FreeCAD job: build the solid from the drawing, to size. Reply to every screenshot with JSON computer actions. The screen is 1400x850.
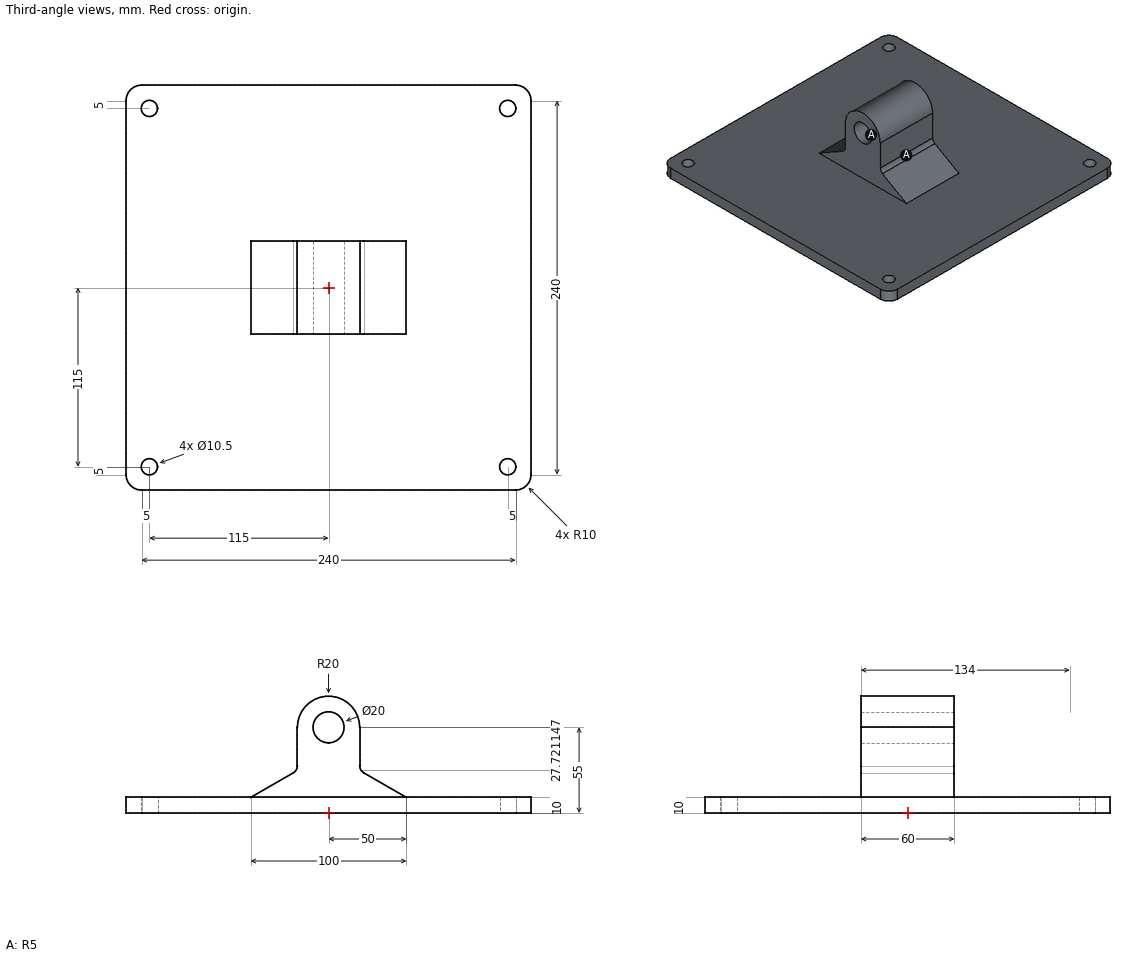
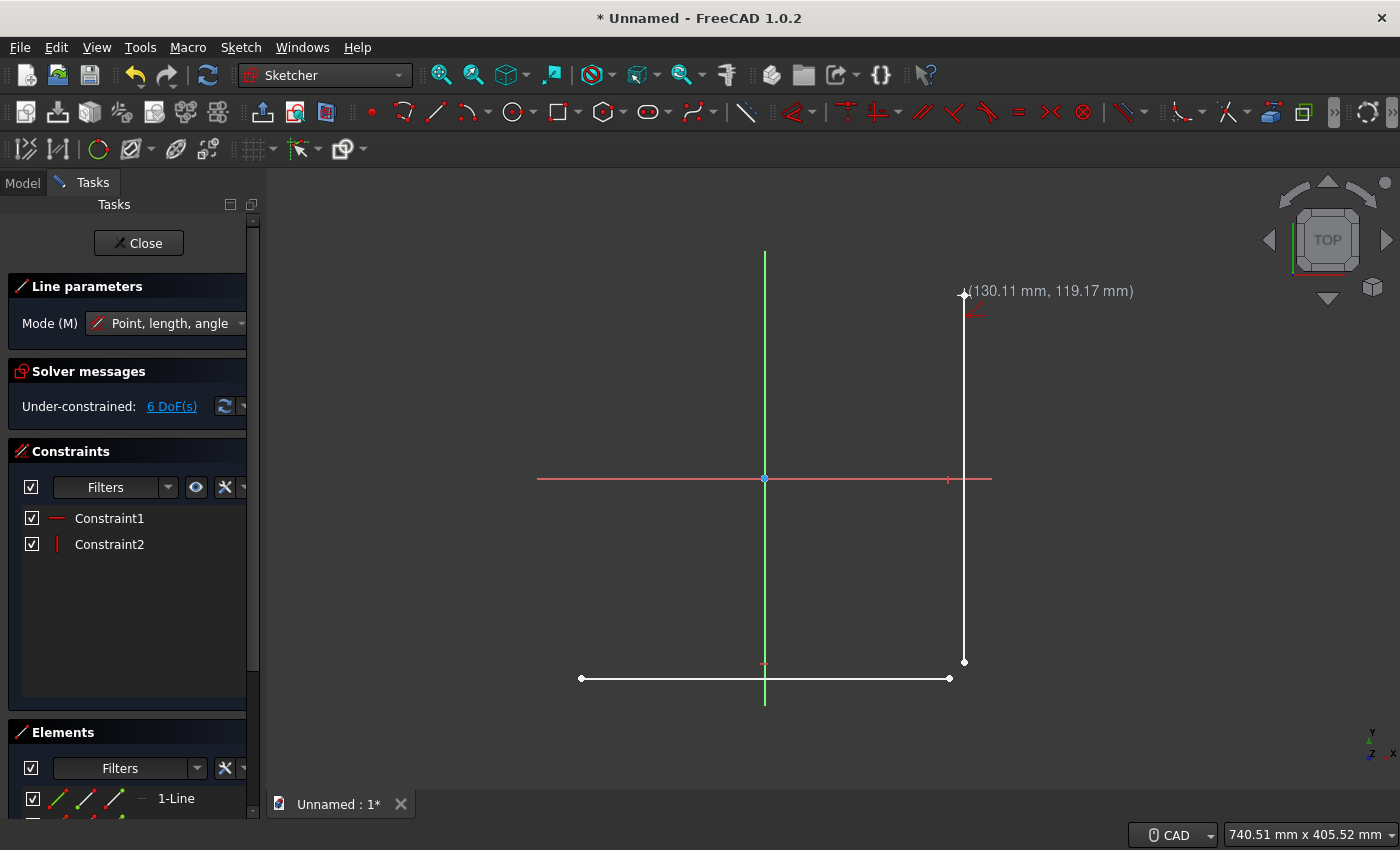
{"action": "left_click", "coordinate": [949, 279]}
{"action": "left_click", "coordinate": [581, 279]}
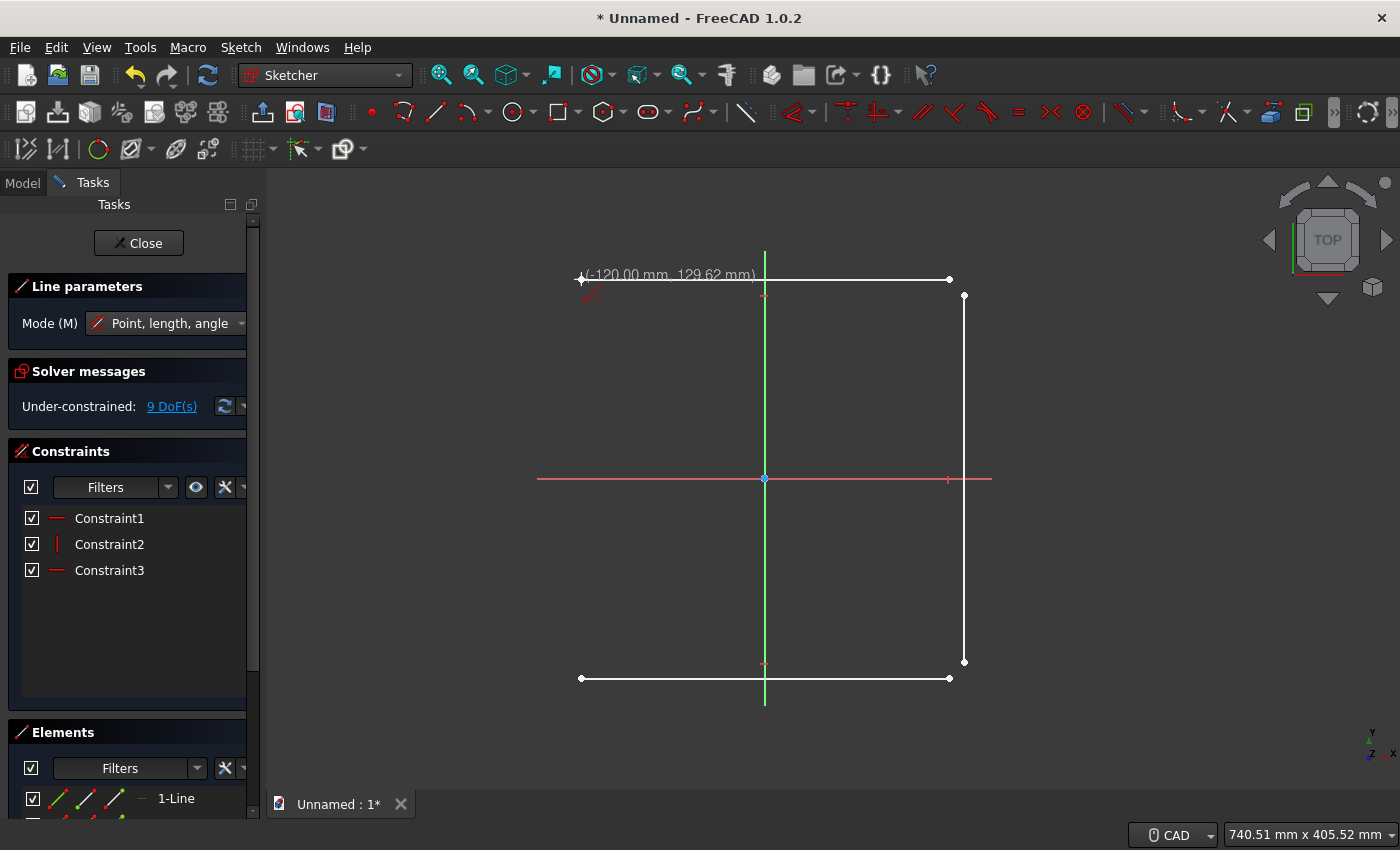
{"action": "left_click", "coordinate": [566, 295]}
{"action": "left_click", "coordinate": [566, 662]}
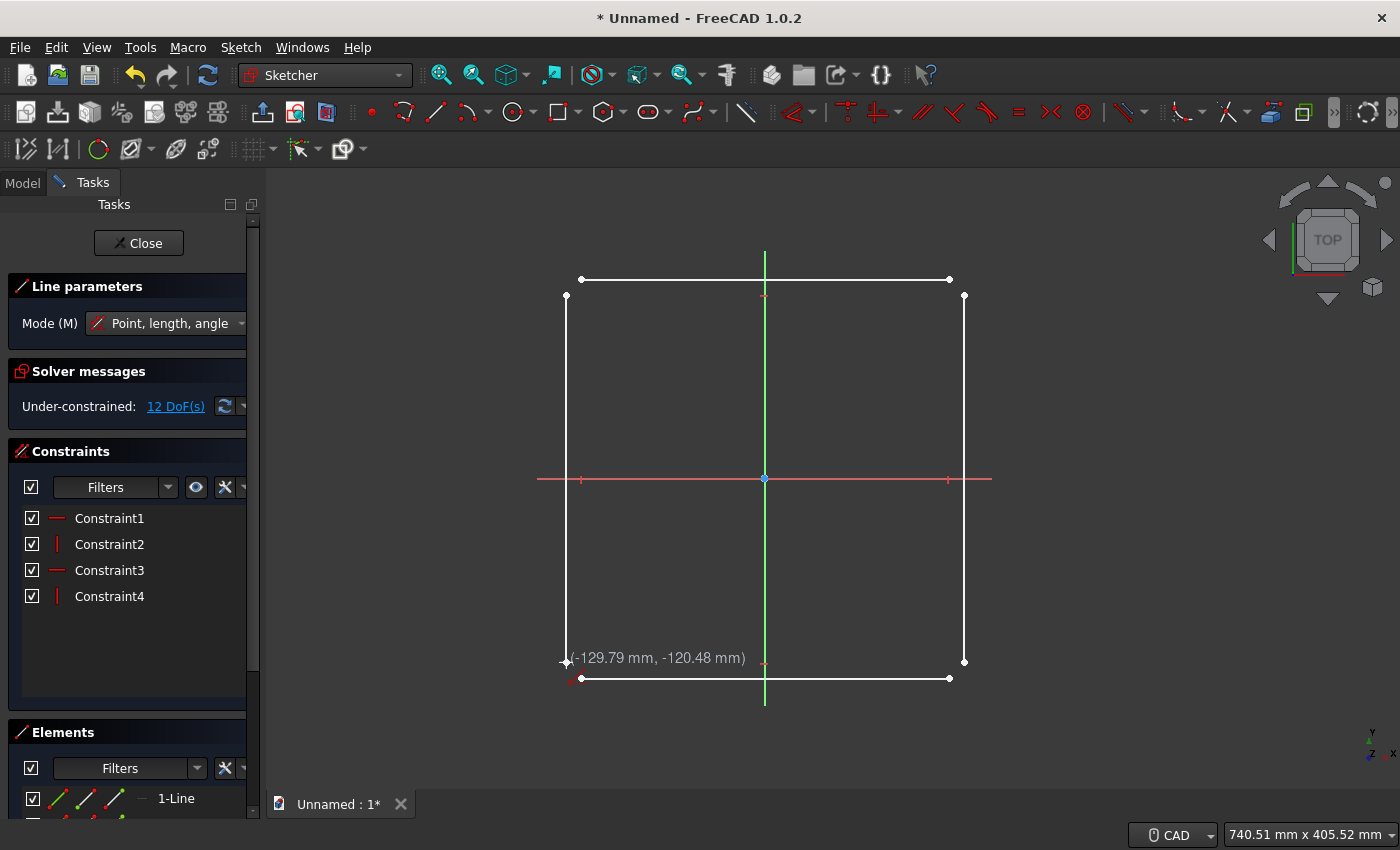
{"action": "left_click", "coordinate": [490, 112]}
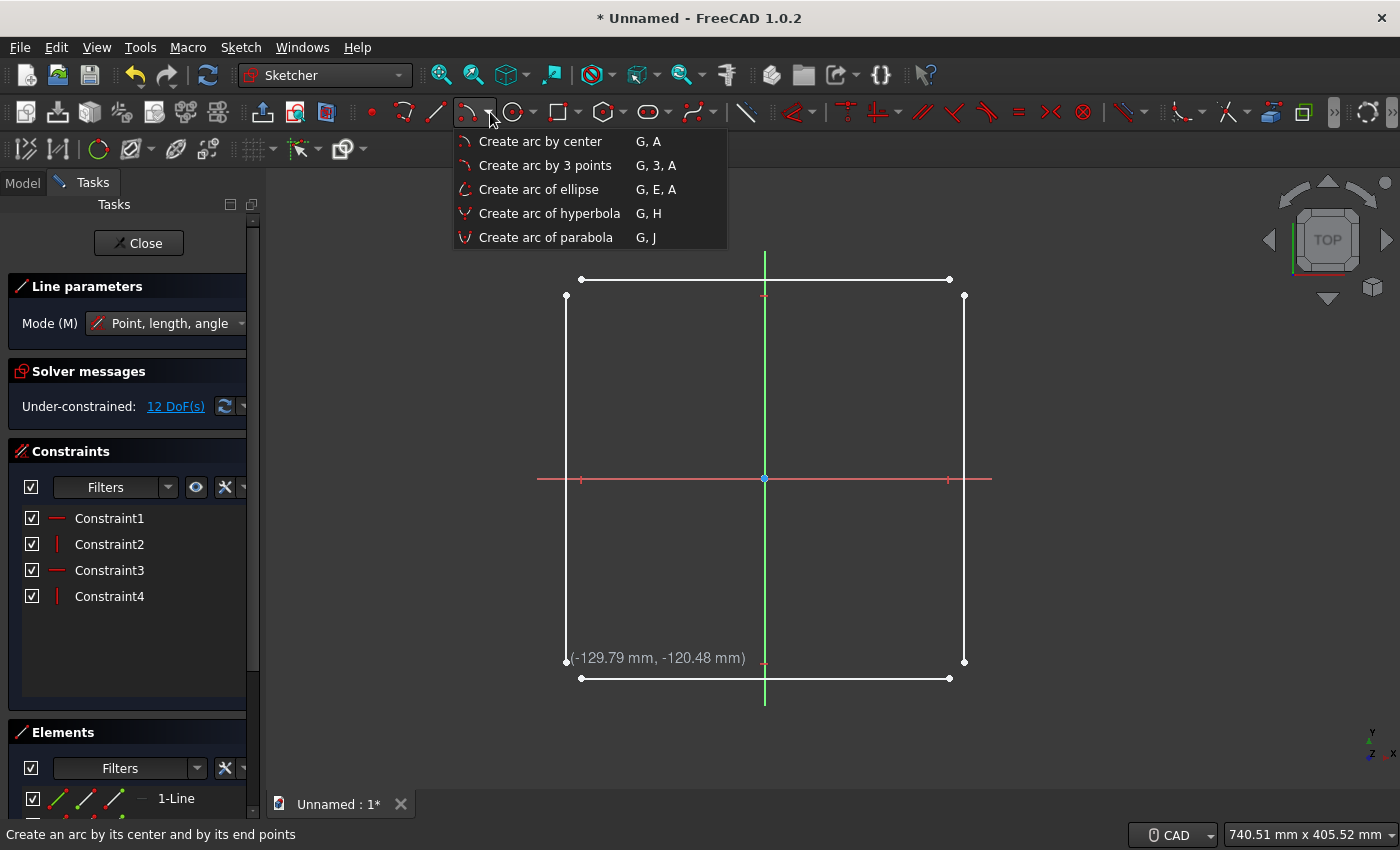
{"action": "left_click", "coordinate": [590, 165]}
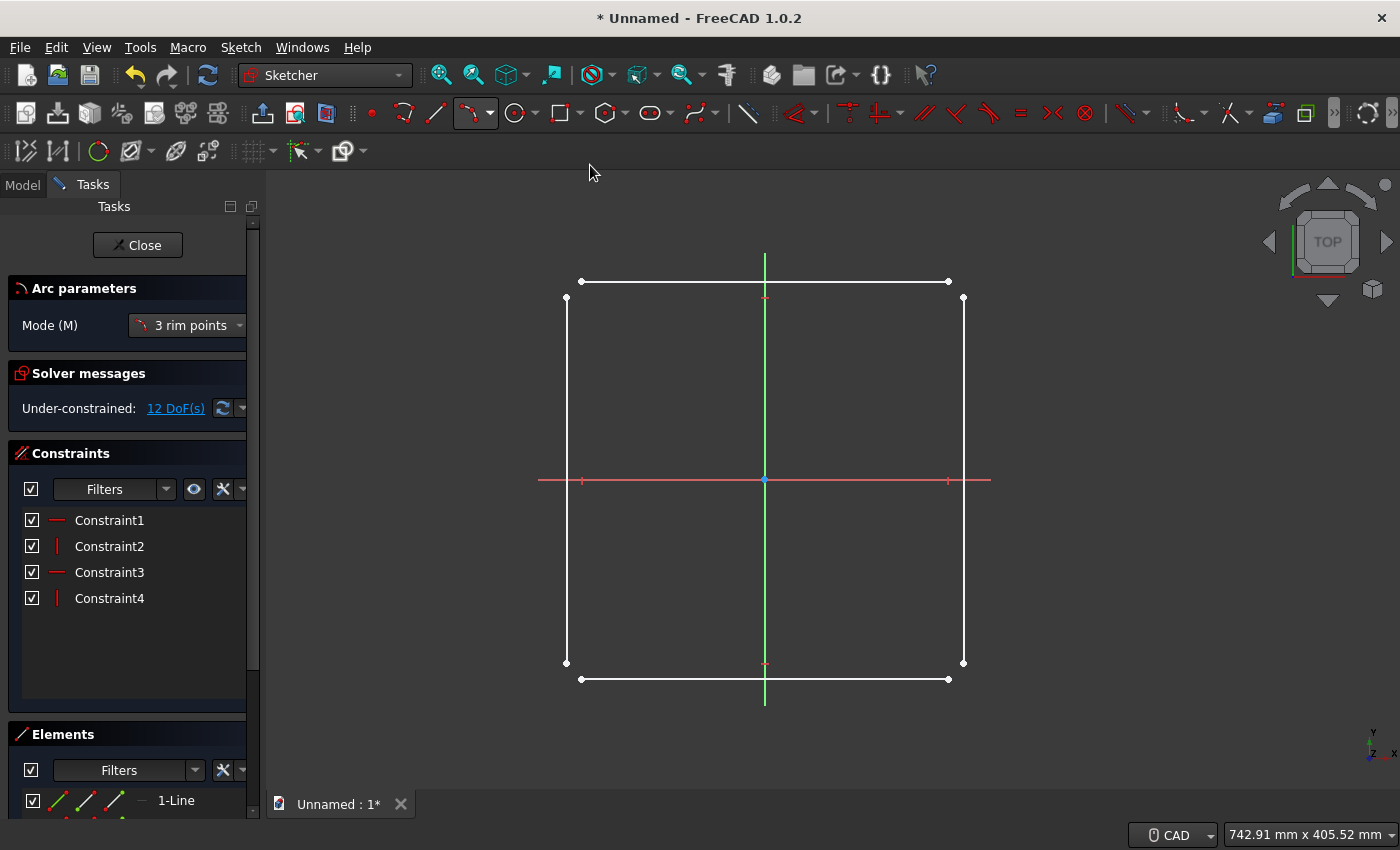
{"action": "left_click", "coordinate": [949, 679]}
{"action": "left_click", "coordinate": [964, 663]}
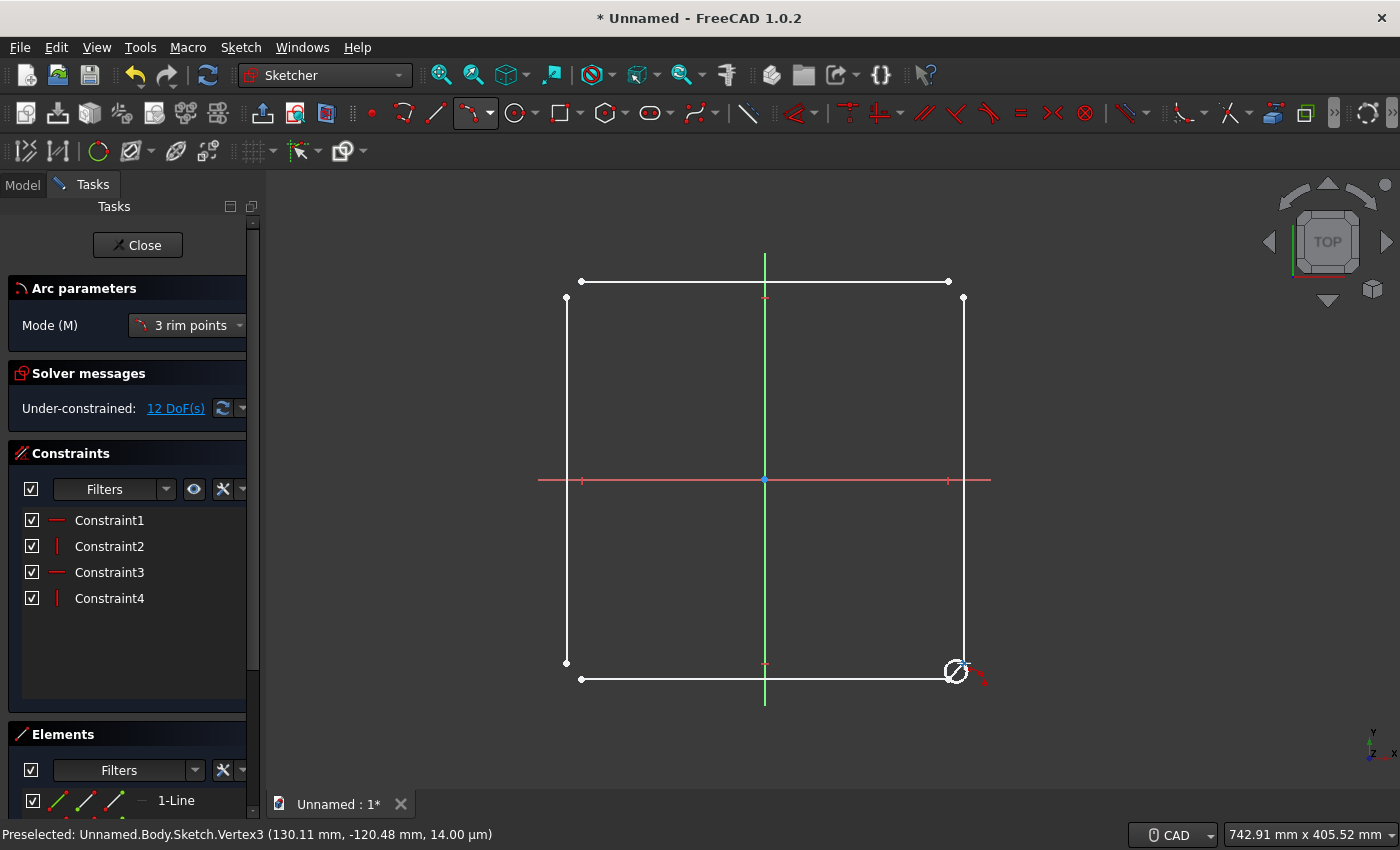
{"action": "scroll", "coordinate": [959, 673], "scroll_direction": "up", "scroll_amount": 7}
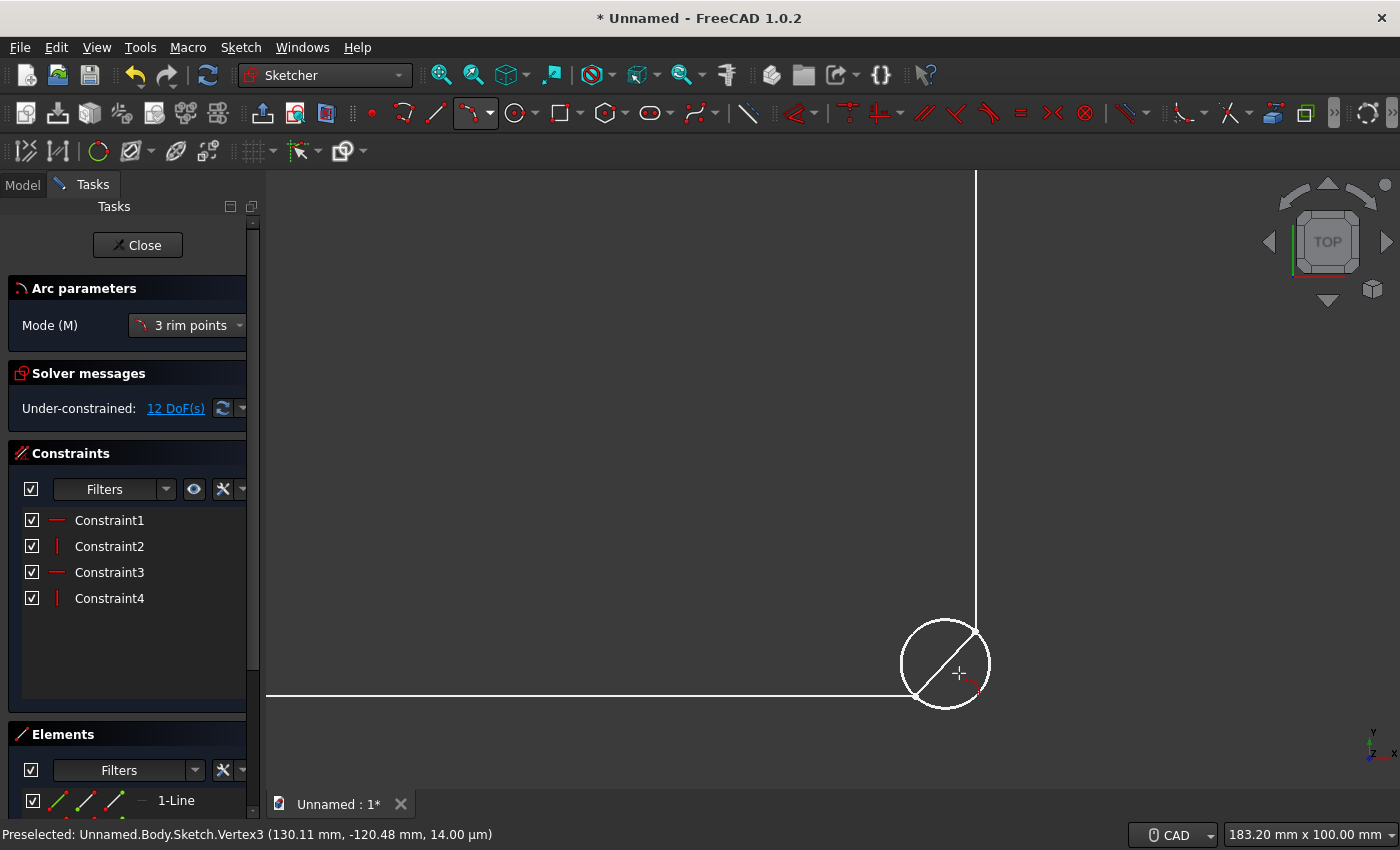
{"action": "left_click", "coordinate": [957, 672]}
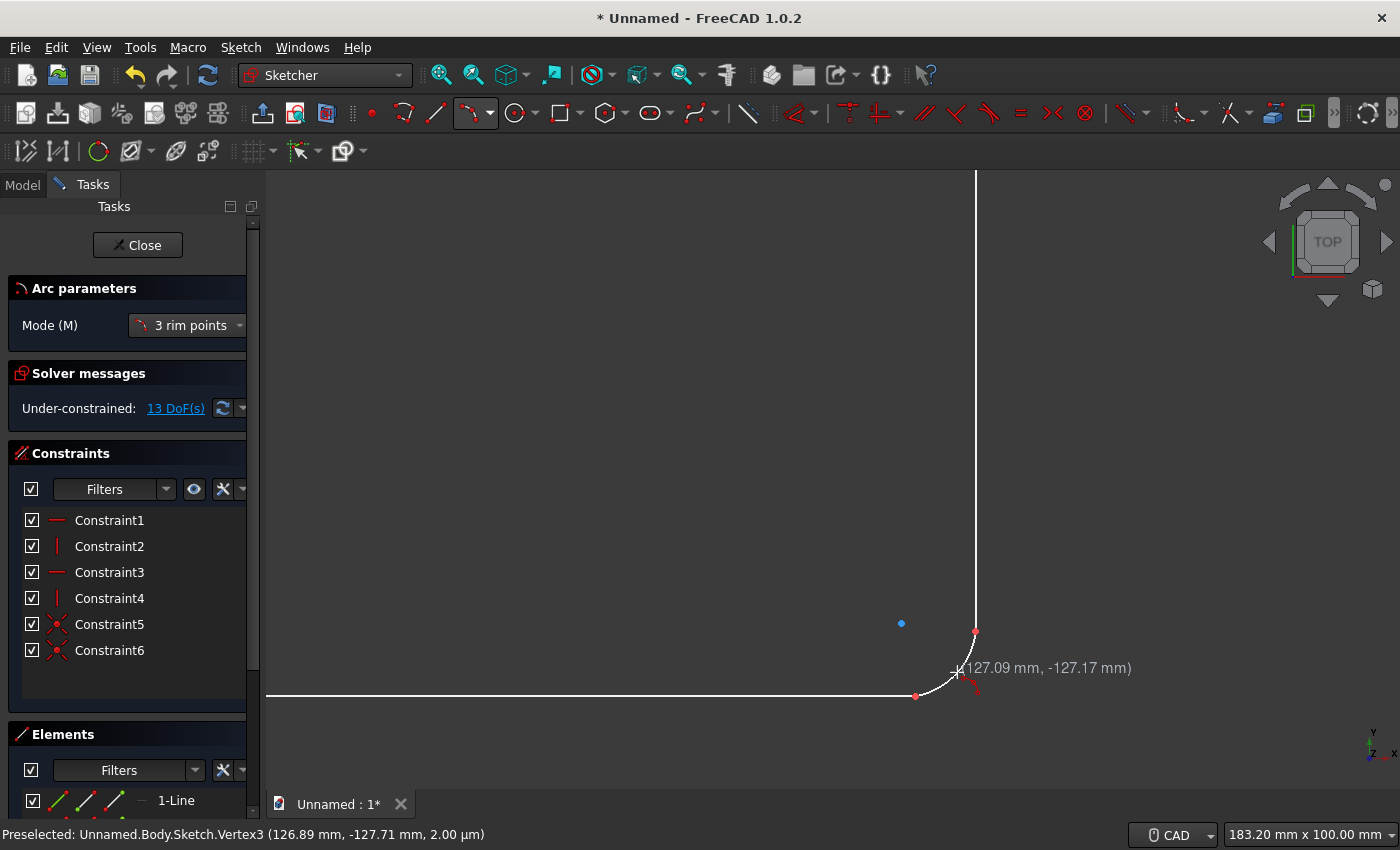
{"action": "scroll", "coordinate": [959, 674], "scroll_direction": "down", "scroll_amount": 7}